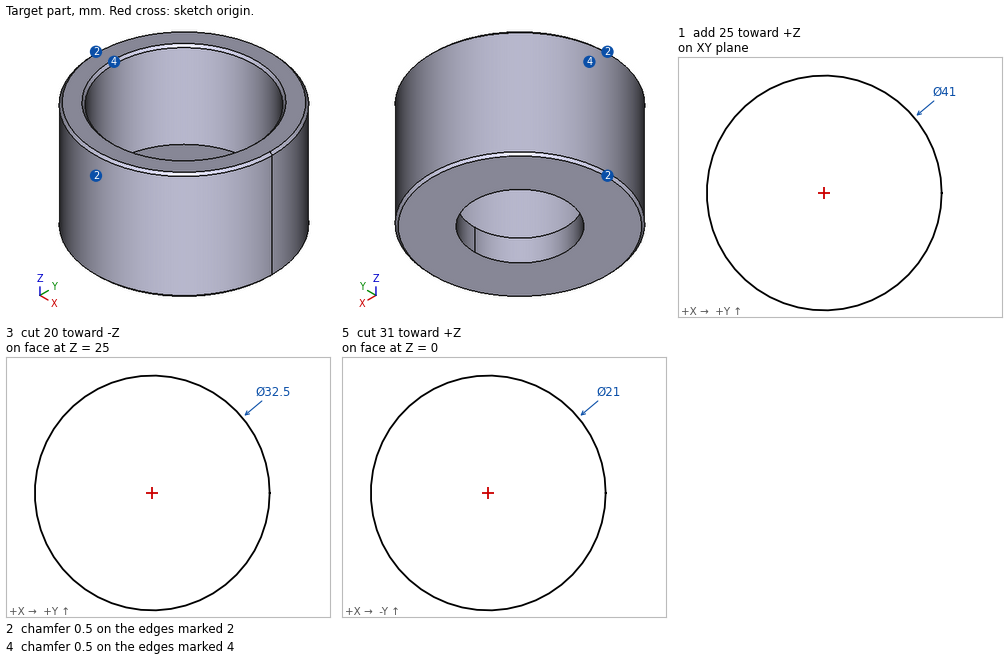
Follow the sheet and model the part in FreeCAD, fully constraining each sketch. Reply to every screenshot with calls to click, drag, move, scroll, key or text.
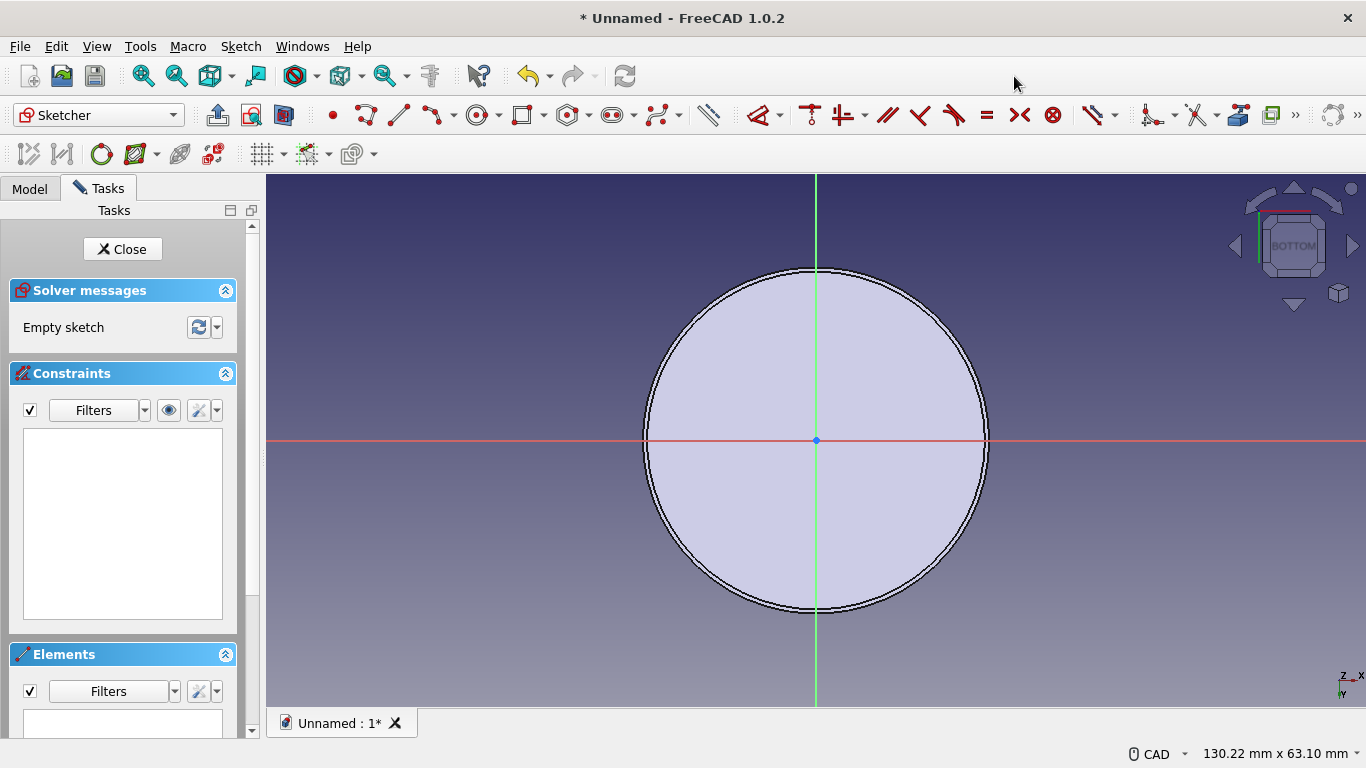
scroll(899, 441, up, 3)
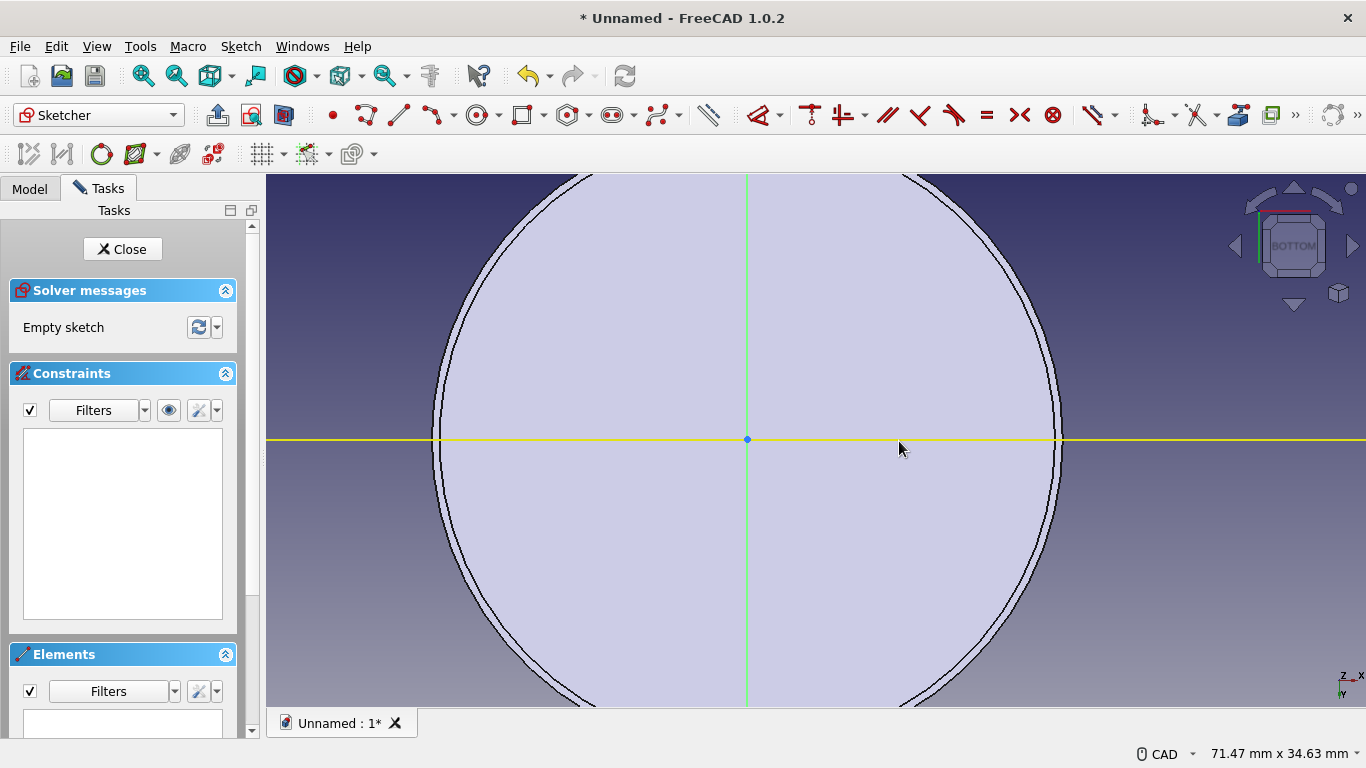
key(g)
key(c)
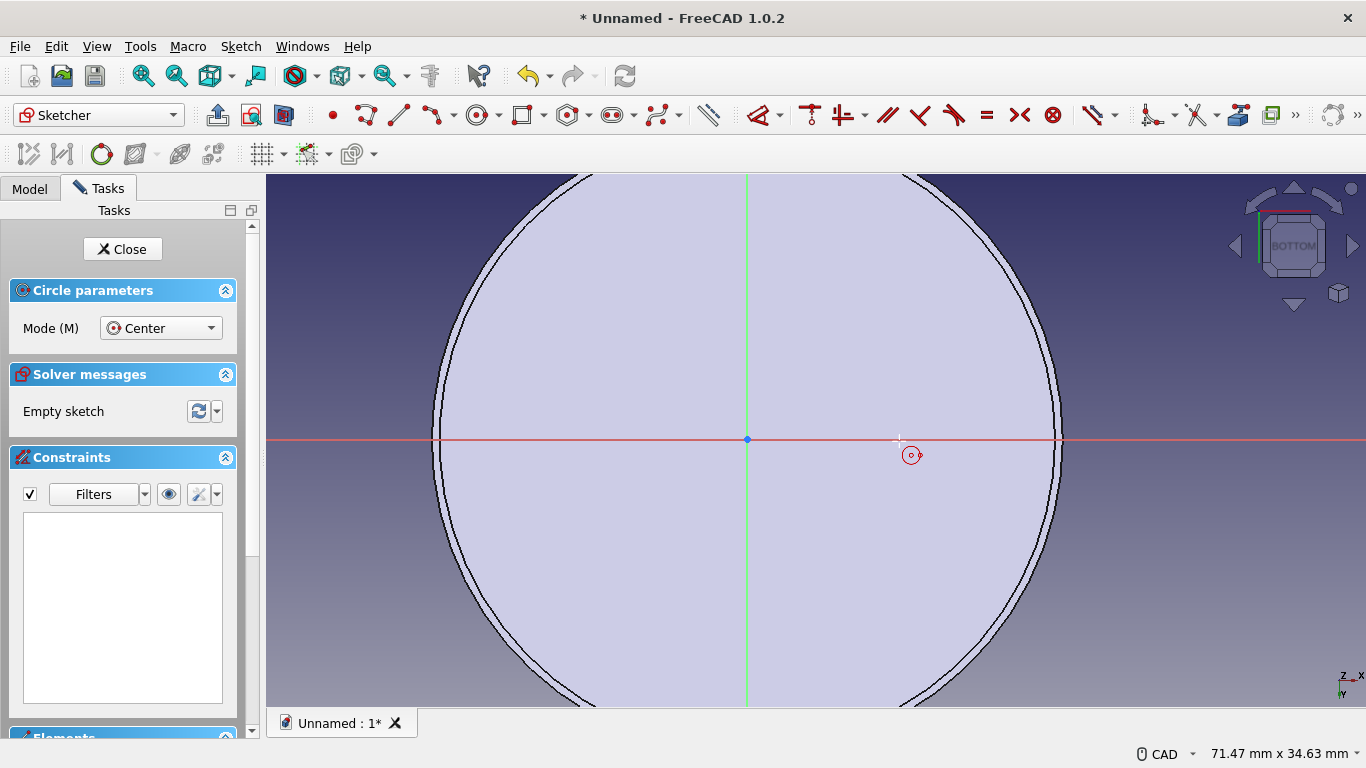
click(747, 440)
move(862, 325)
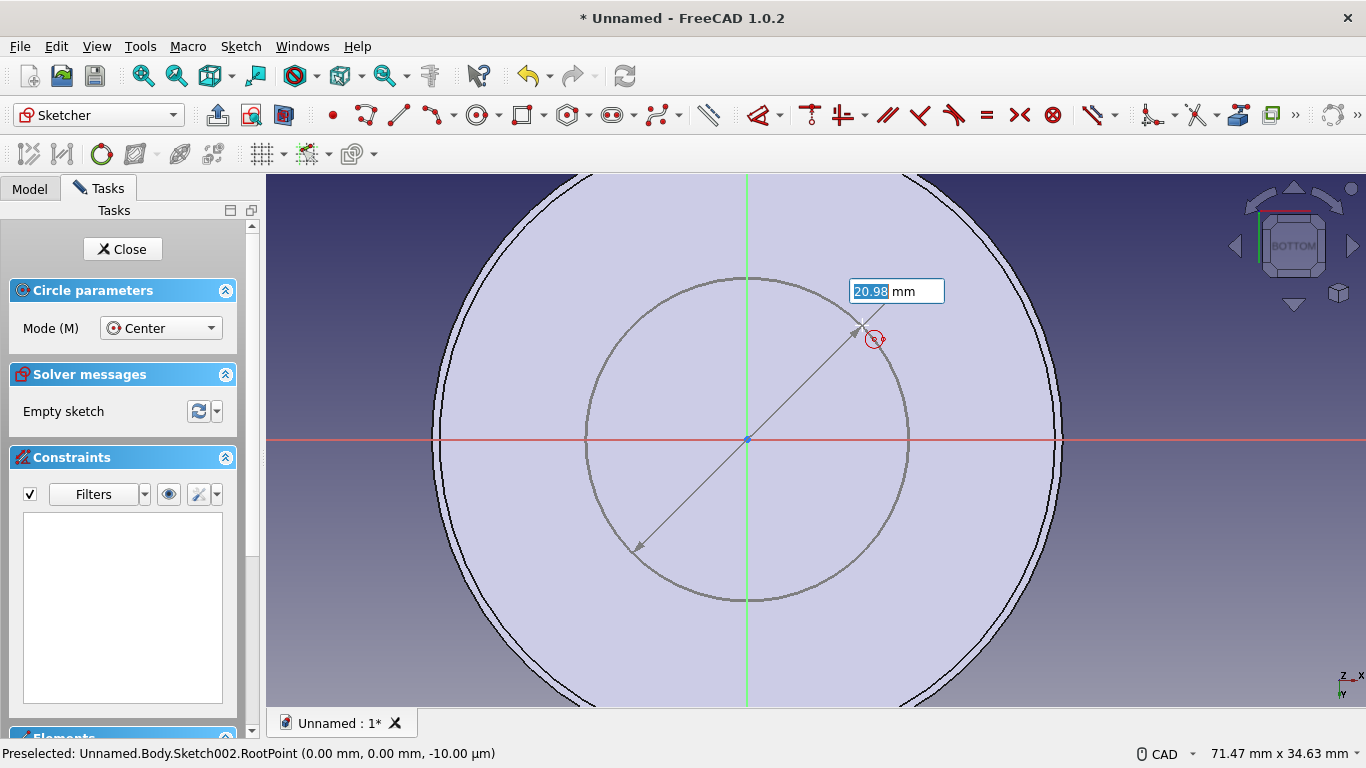
text(21)
key(Return)
key(Escape)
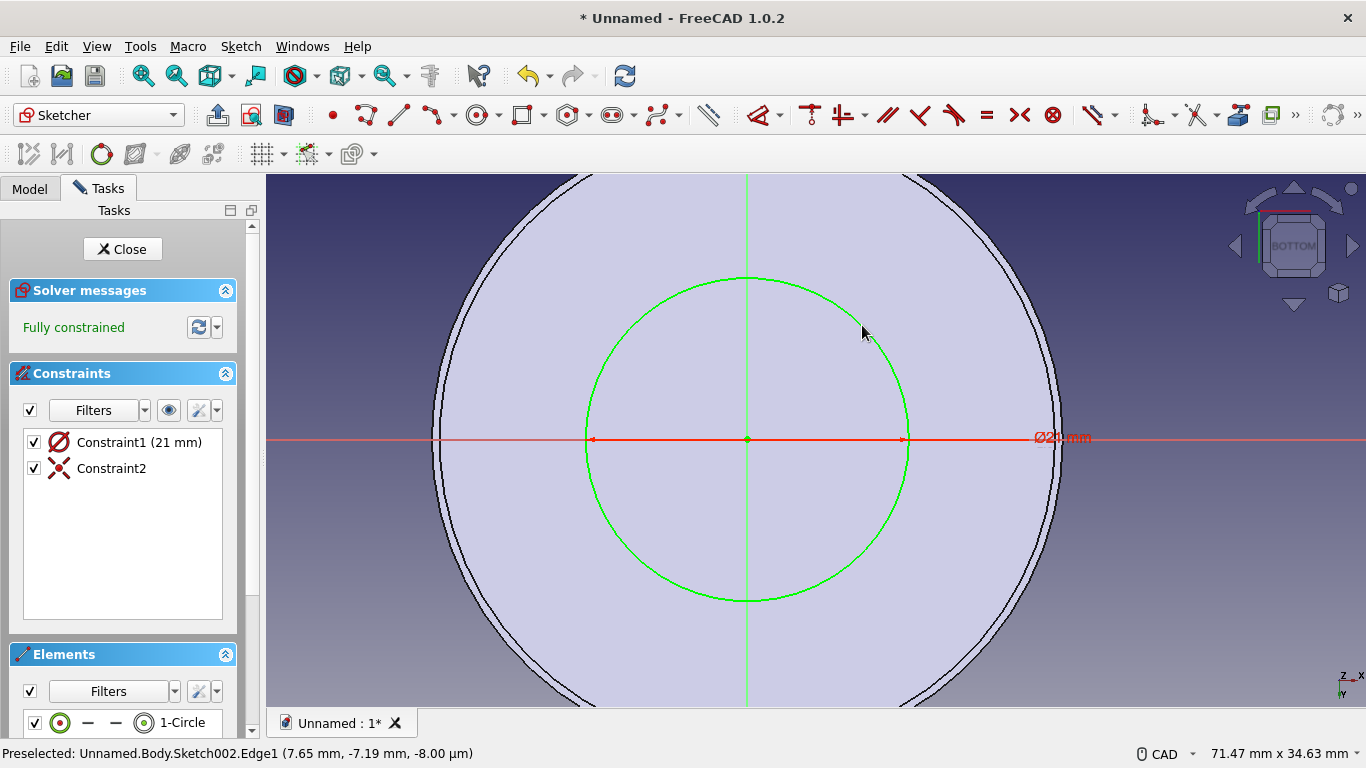
click(123, 249)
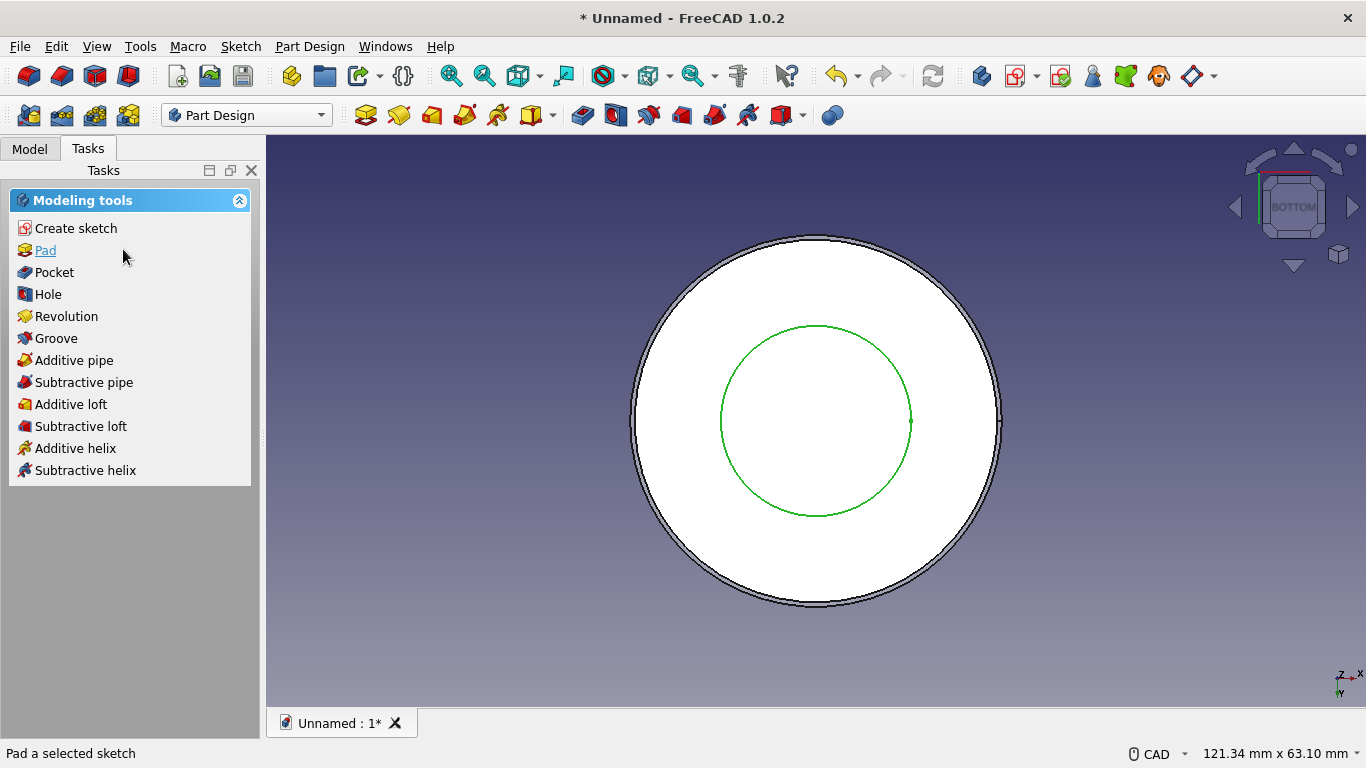
click(583, 116)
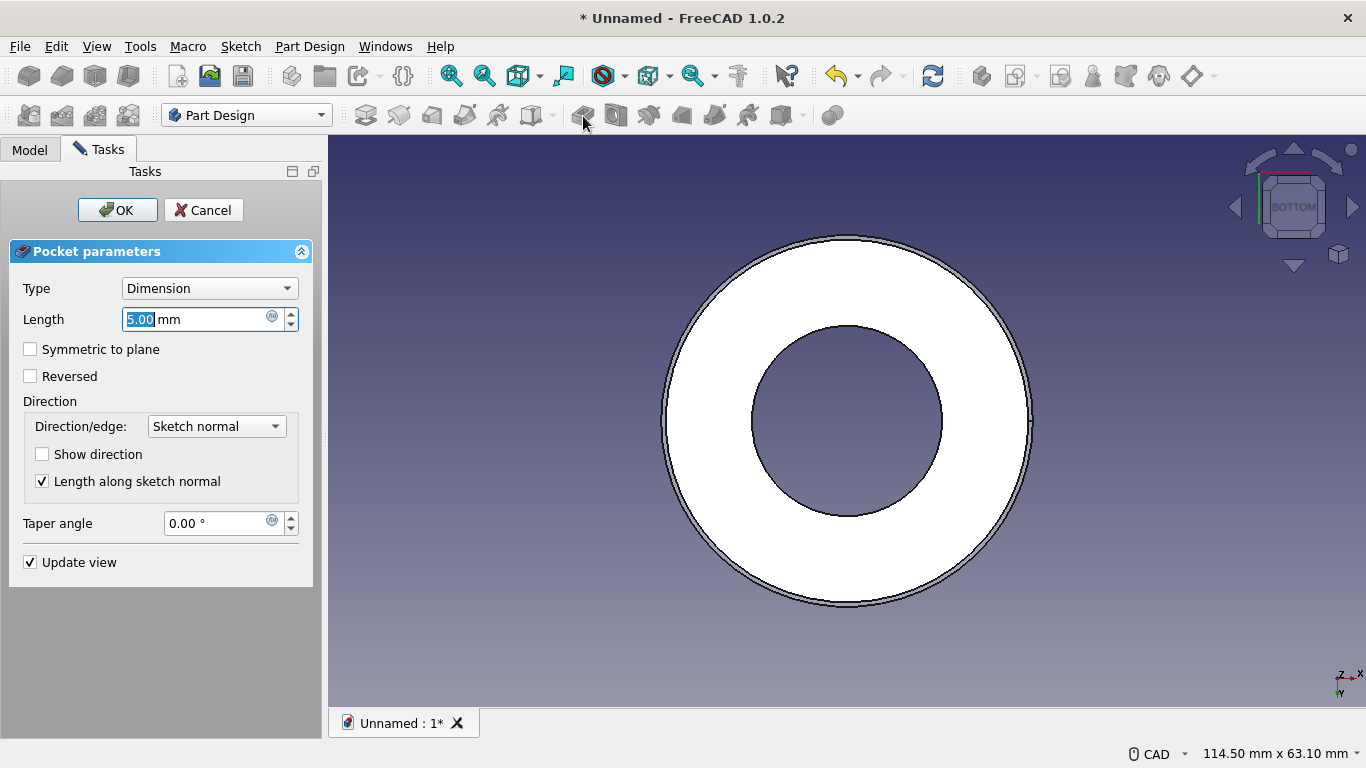
text(31)
key(Tab)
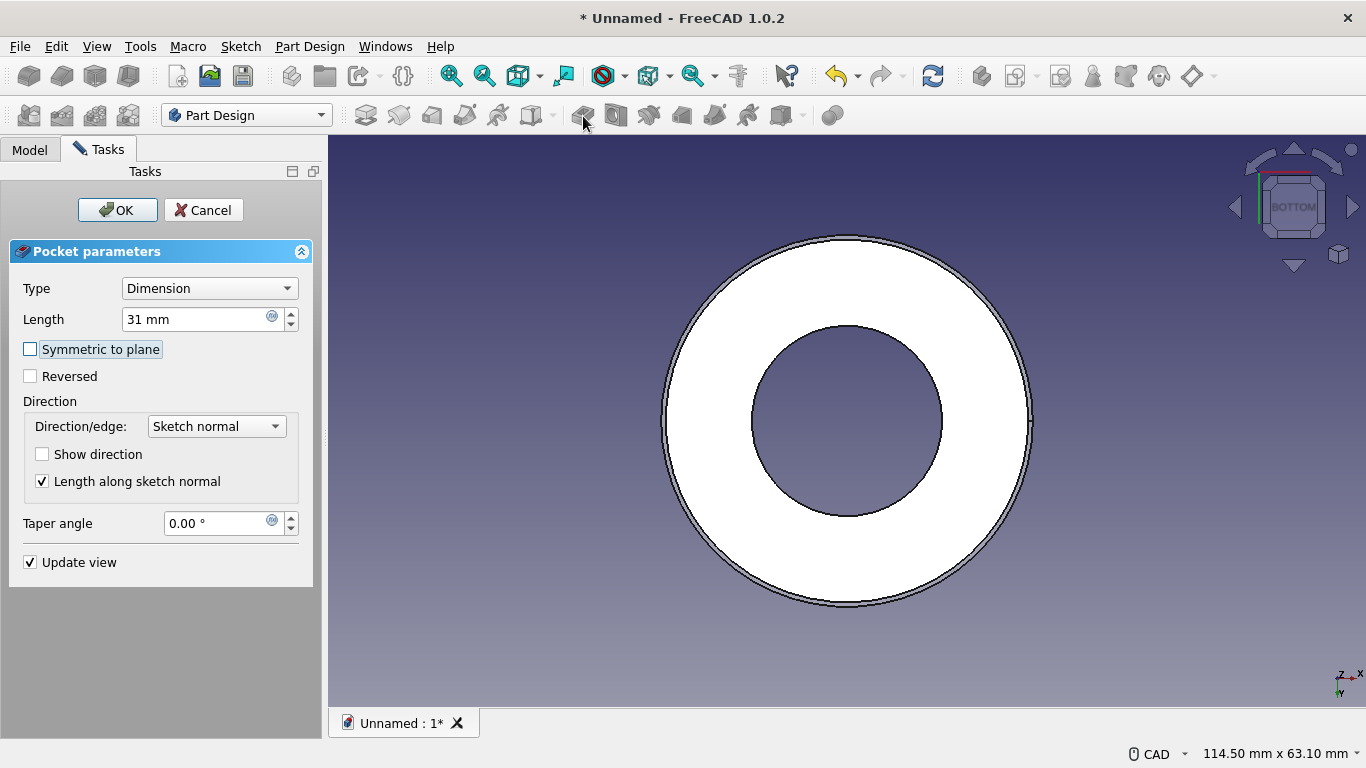
click(118, 210)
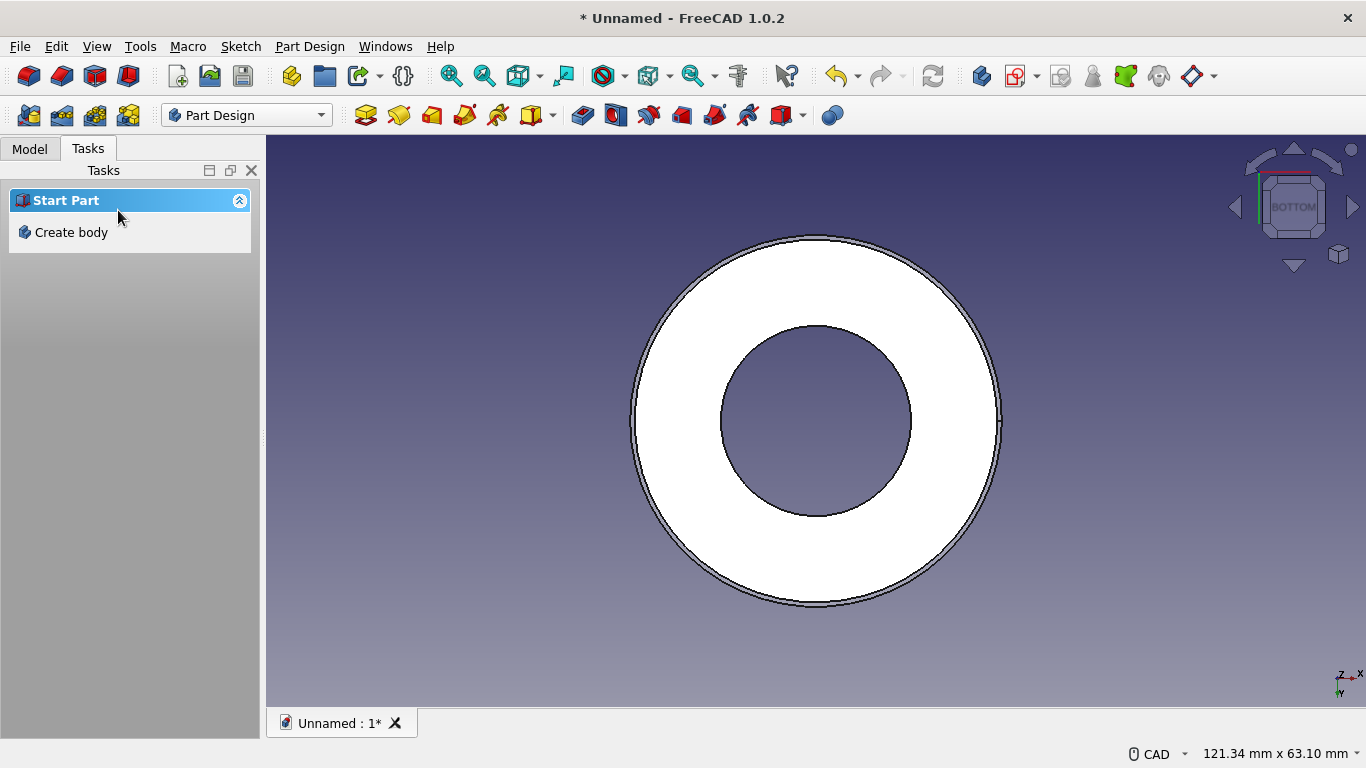
key(0)